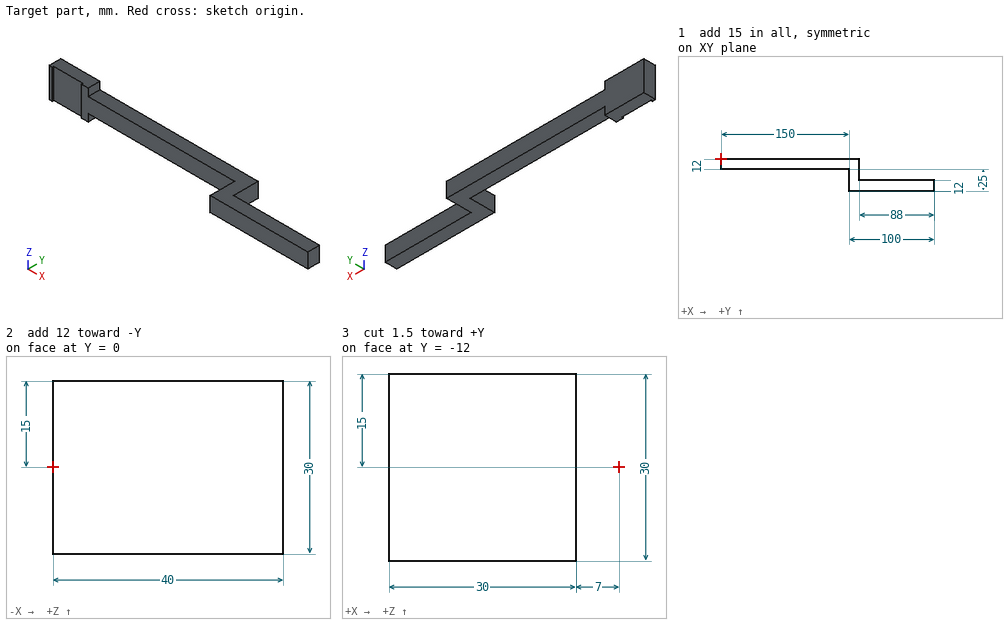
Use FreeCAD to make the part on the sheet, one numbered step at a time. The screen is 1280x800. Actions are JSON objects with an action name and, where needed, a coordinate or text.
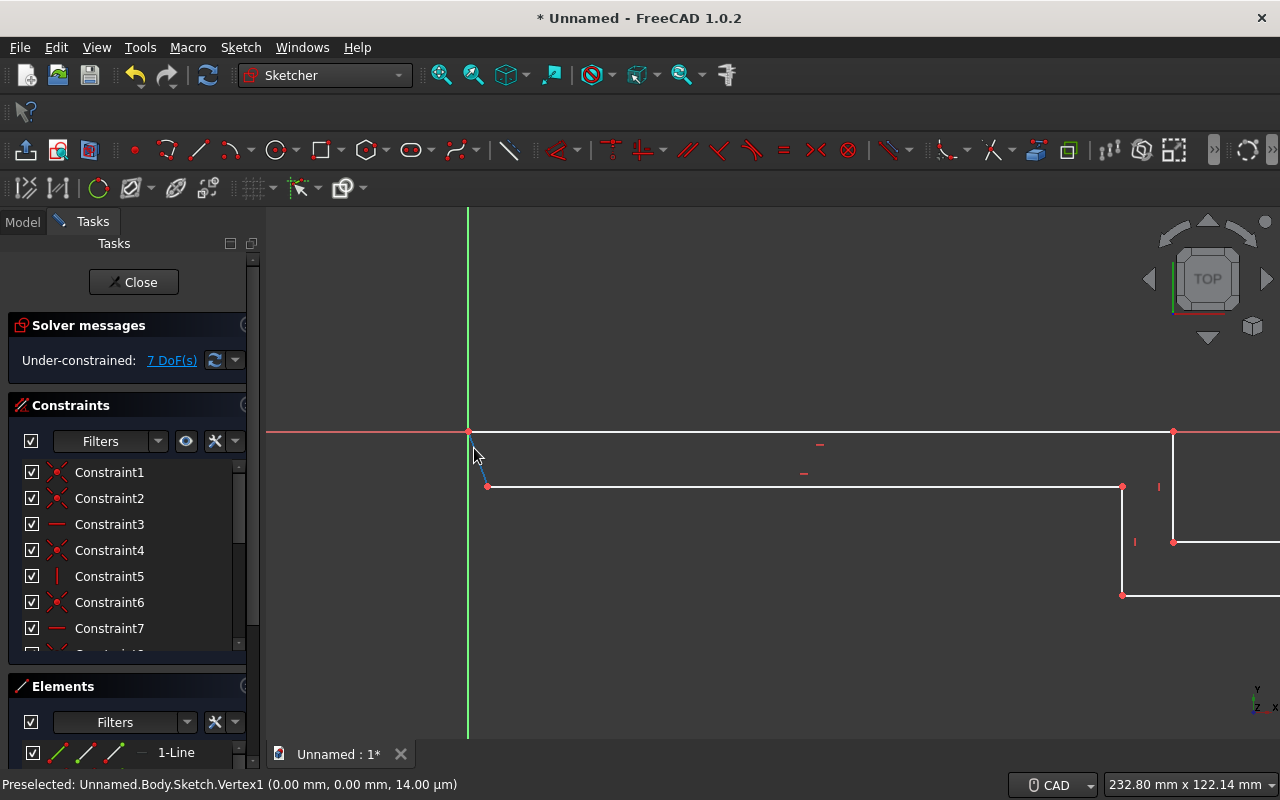
{"action": "left_click", "coordinate": [474, 448]}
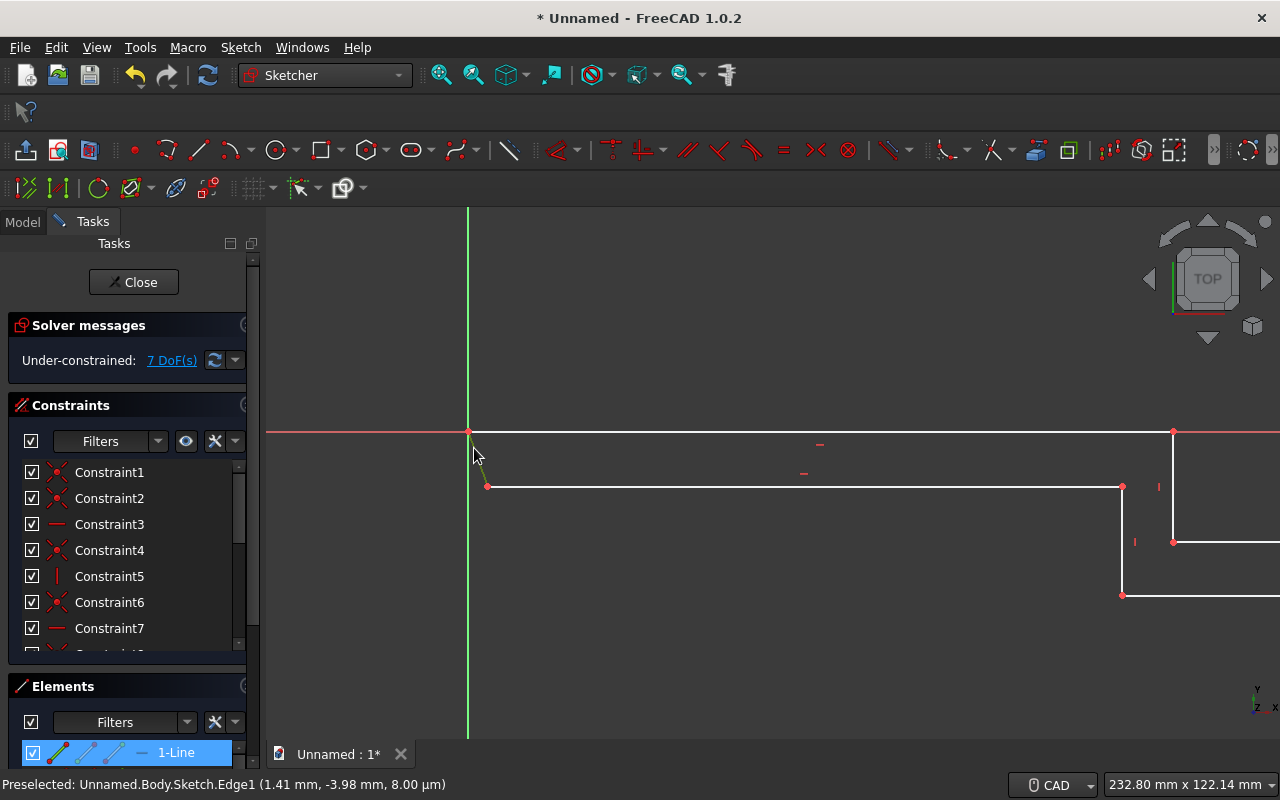
{"action": "left_click", "coordinate": [666, 150]}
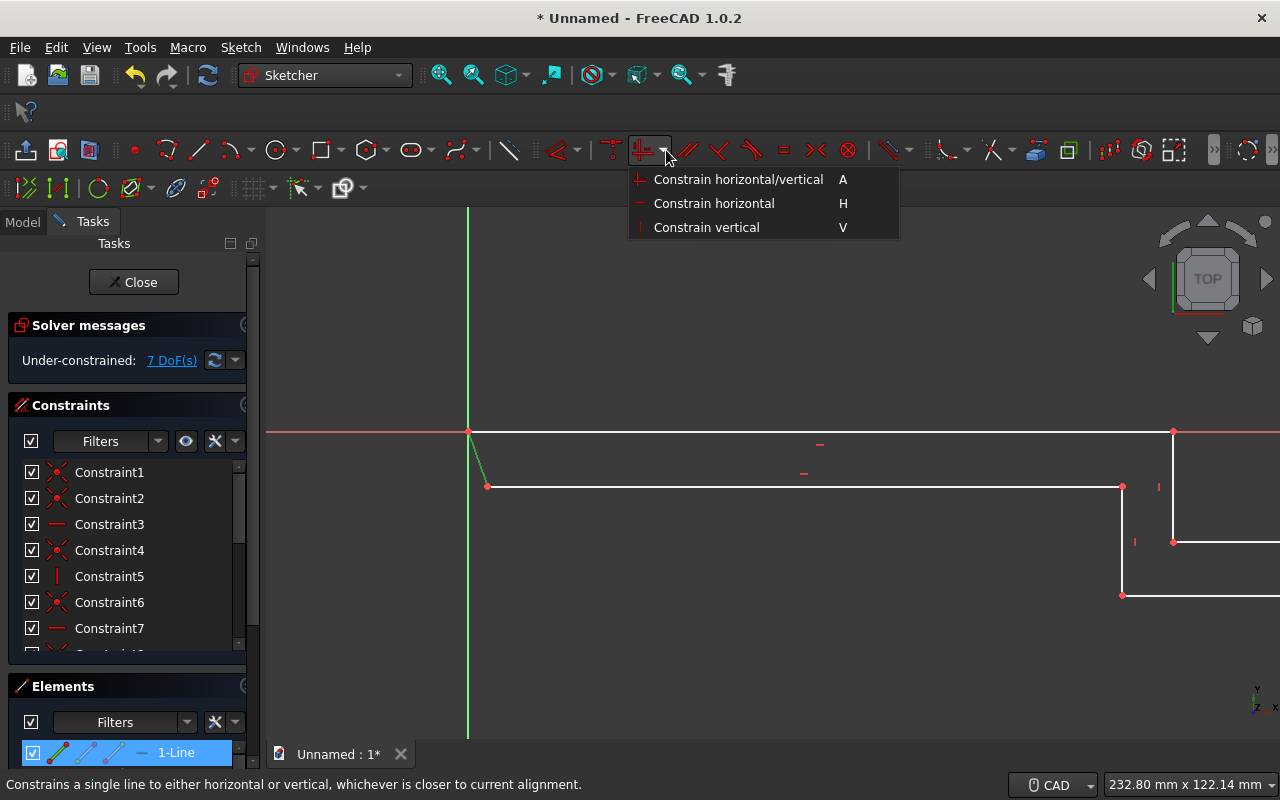
{"action": "left_click", "coordinate": [764, 227]}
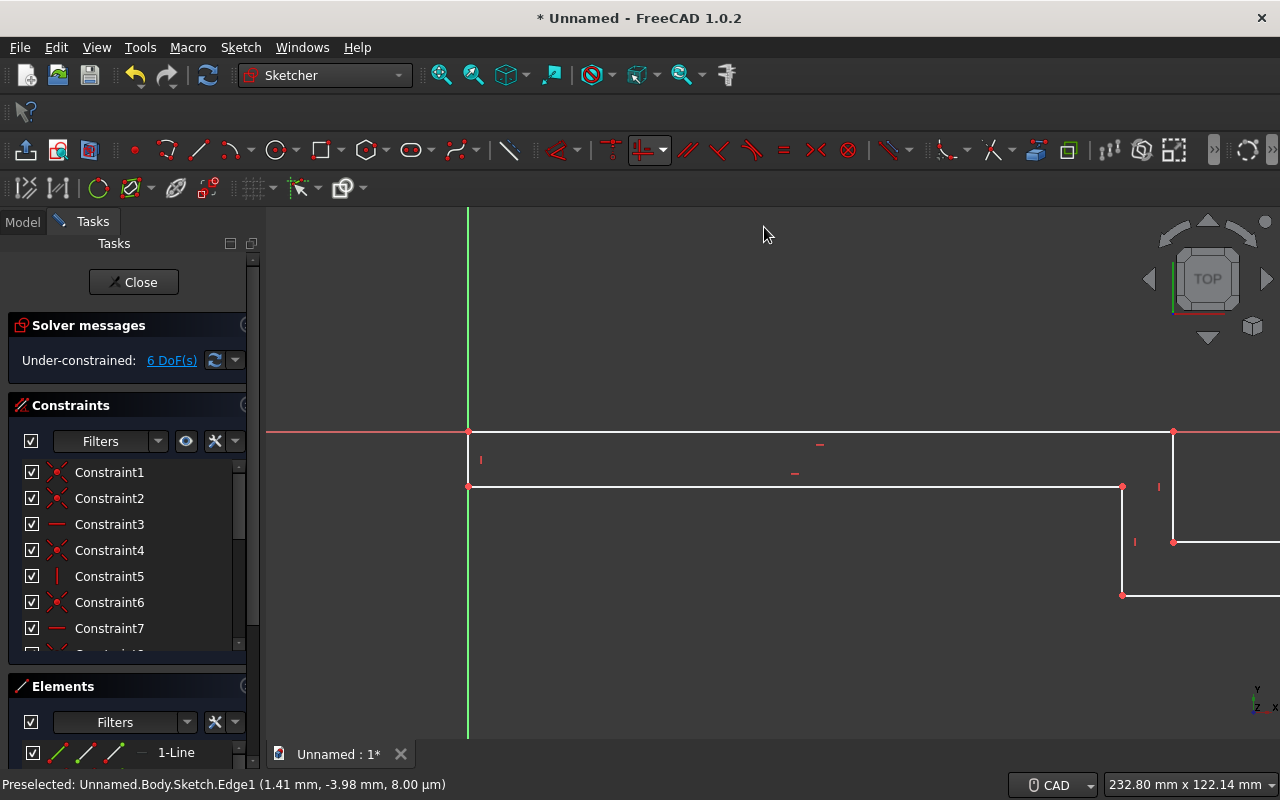
{"action": "left_click", "coordinate": [468, 448]}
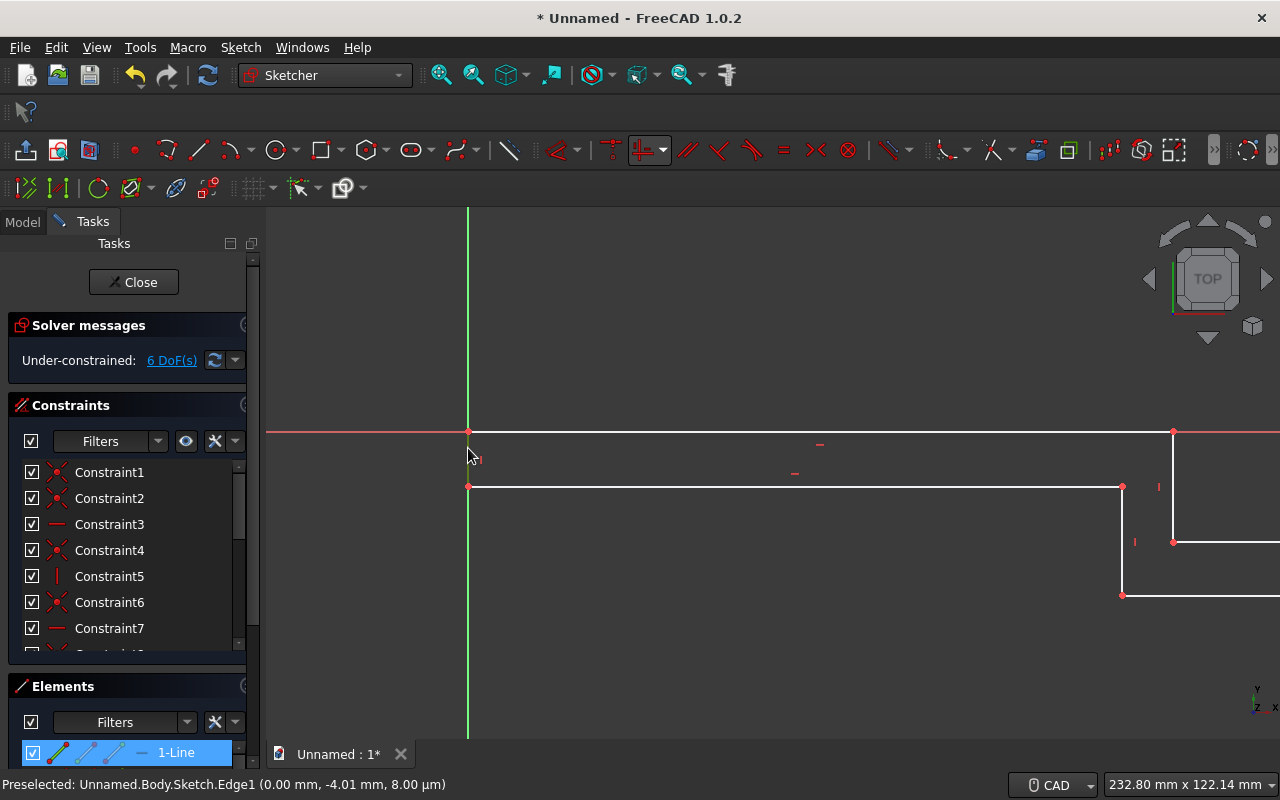
{"action": "key", "text": "i"}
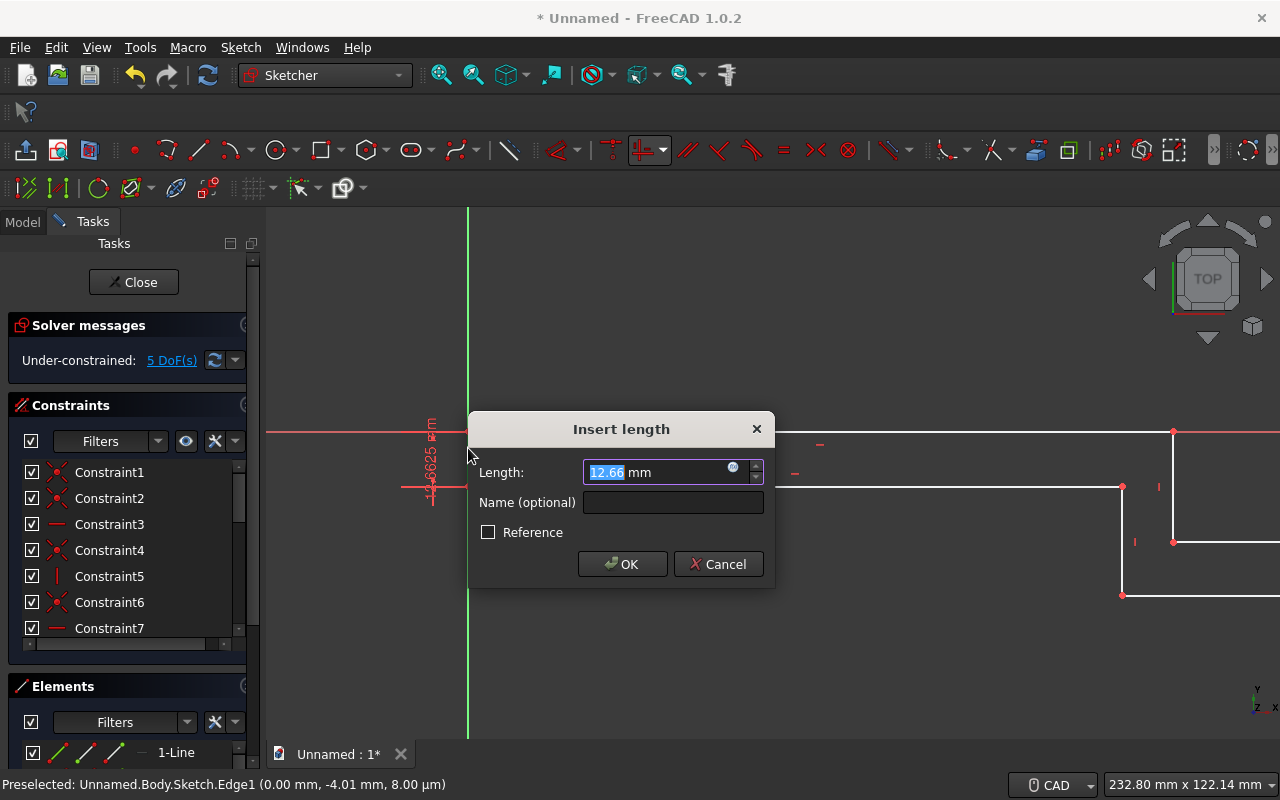
{"action": "type", "text": "12"}
{"action": "key", "text": "Return"}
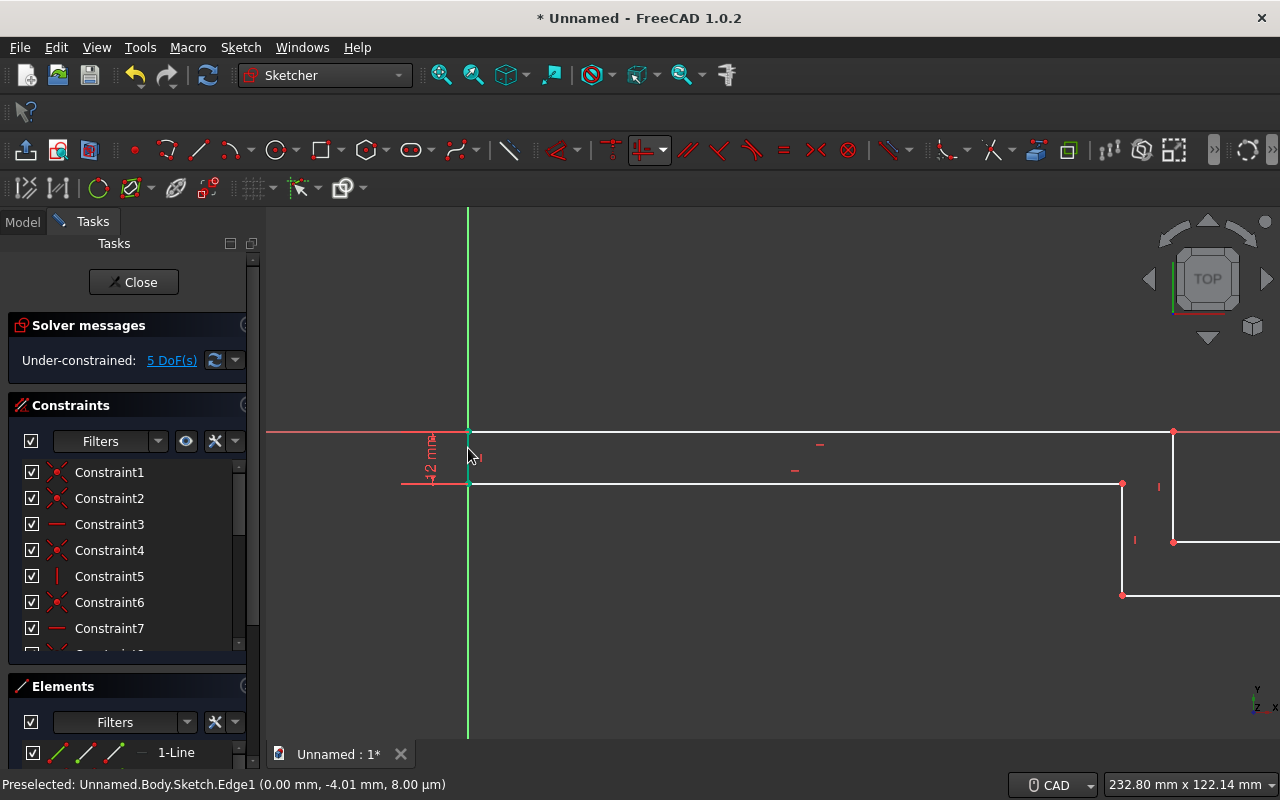
{"action": "scroll", "coordinate": [330, 425], "scroll_direction": "down", "scroll_amount": 3}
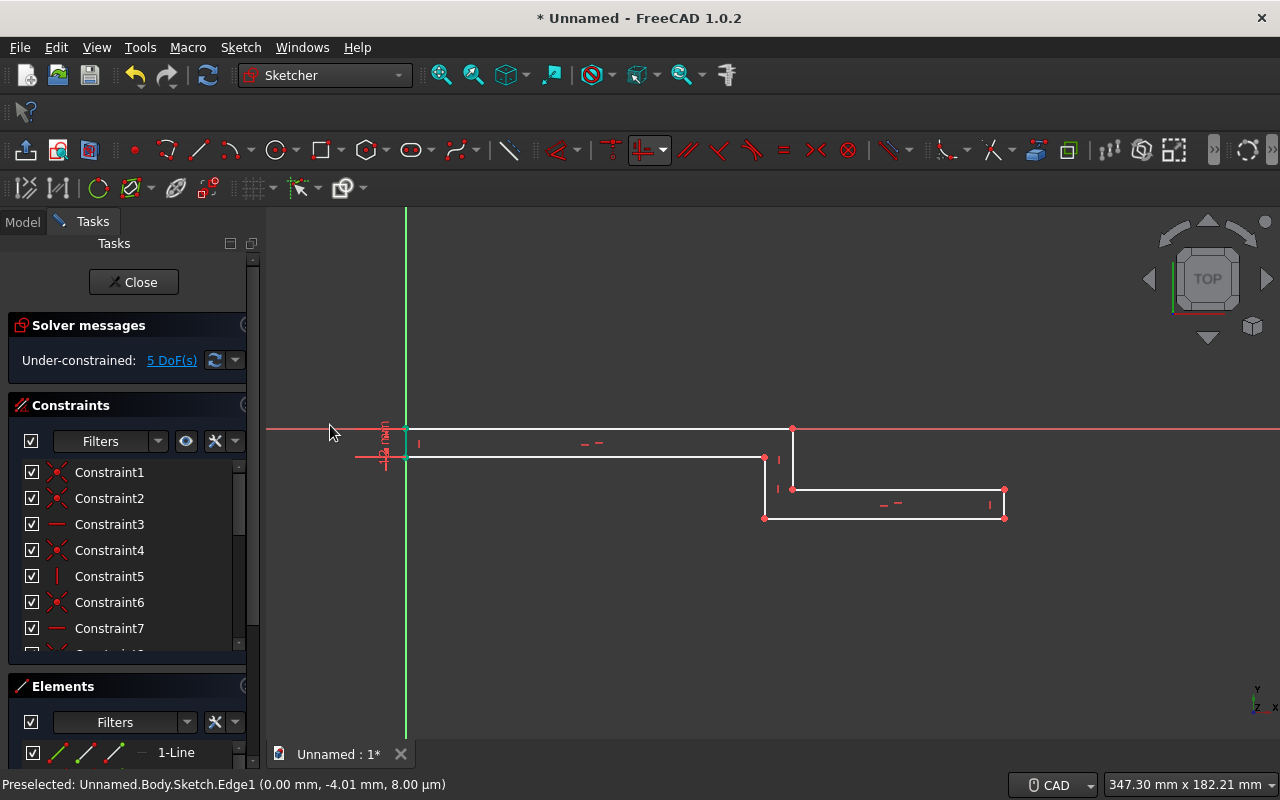
{"action": "left_click", "coordinate": [765, 476]}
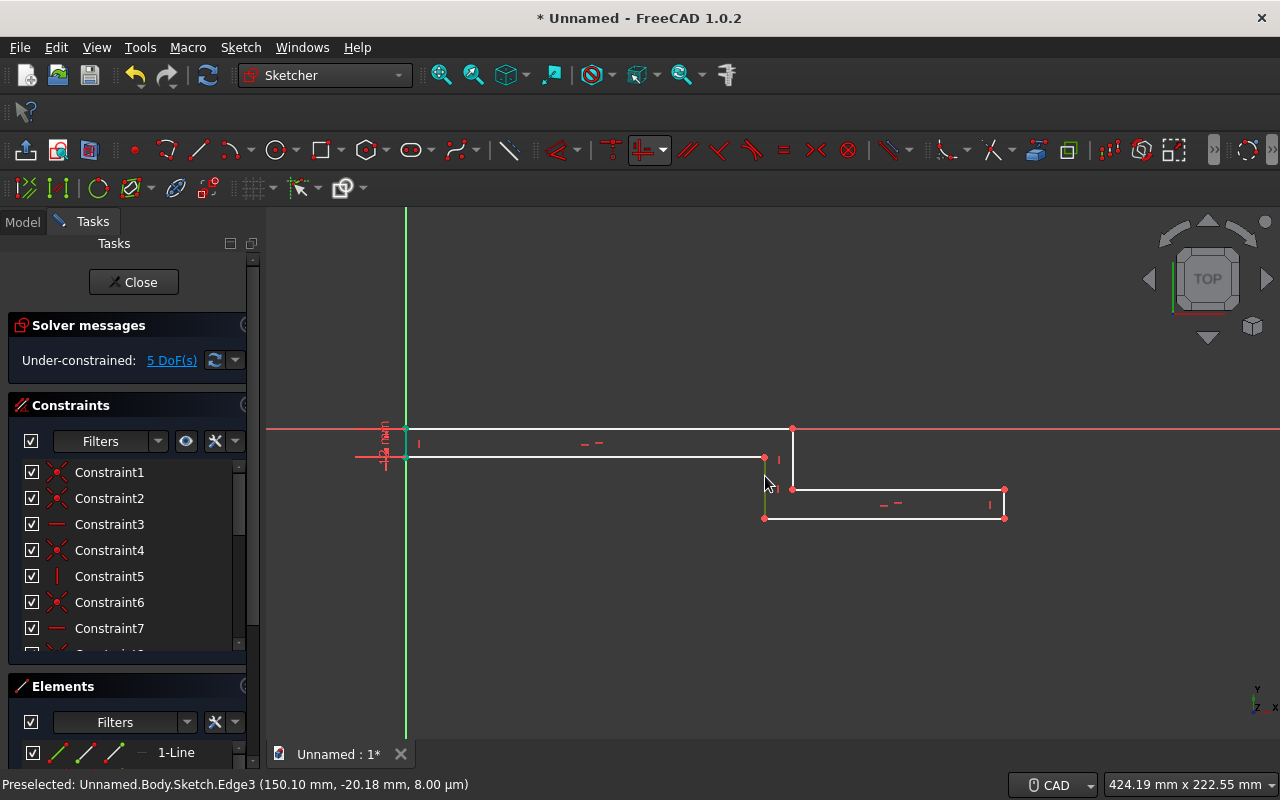
{"action": "key", "text": "i"}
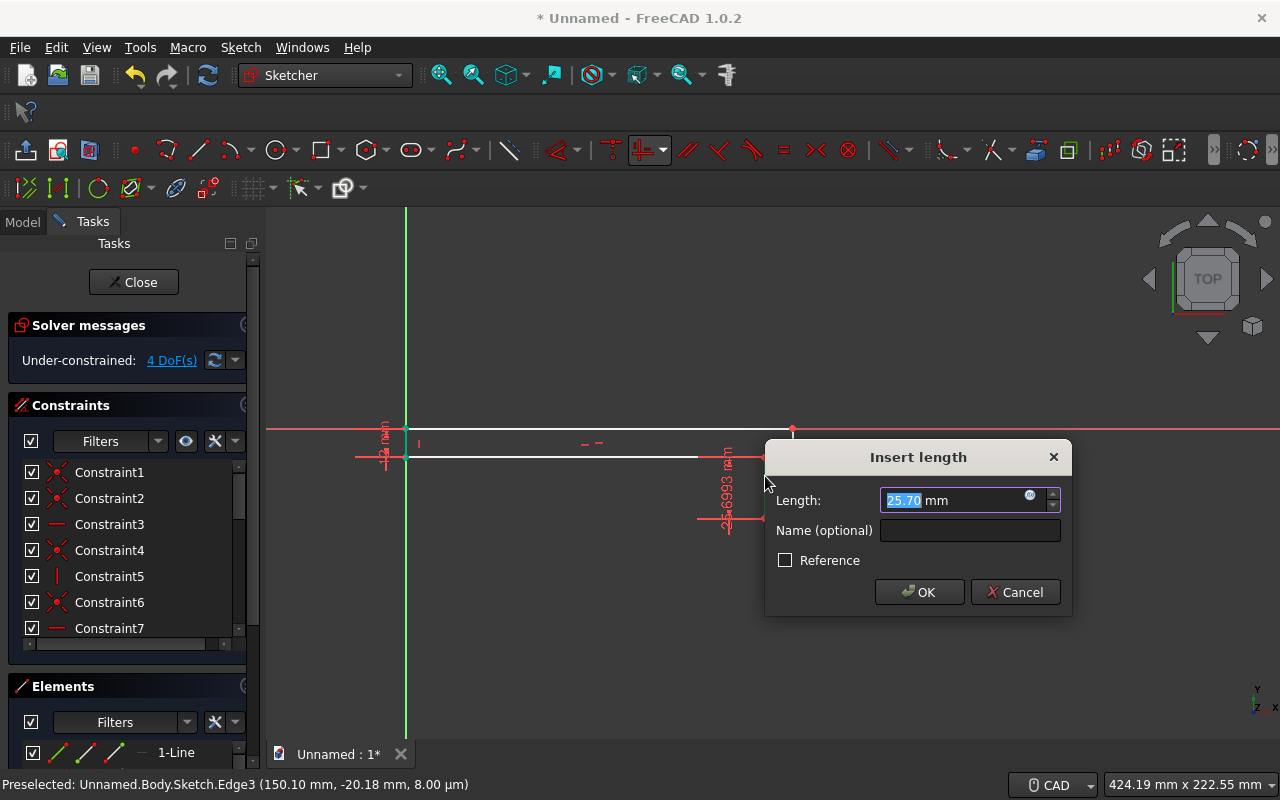
{"action": "type", "text": "25"}
{"action": "key", "text": "Return"}